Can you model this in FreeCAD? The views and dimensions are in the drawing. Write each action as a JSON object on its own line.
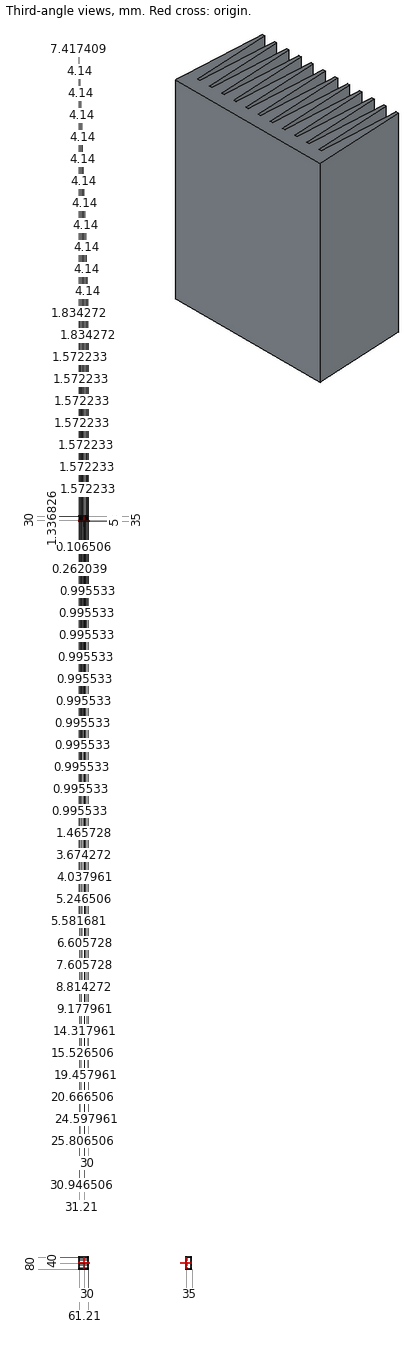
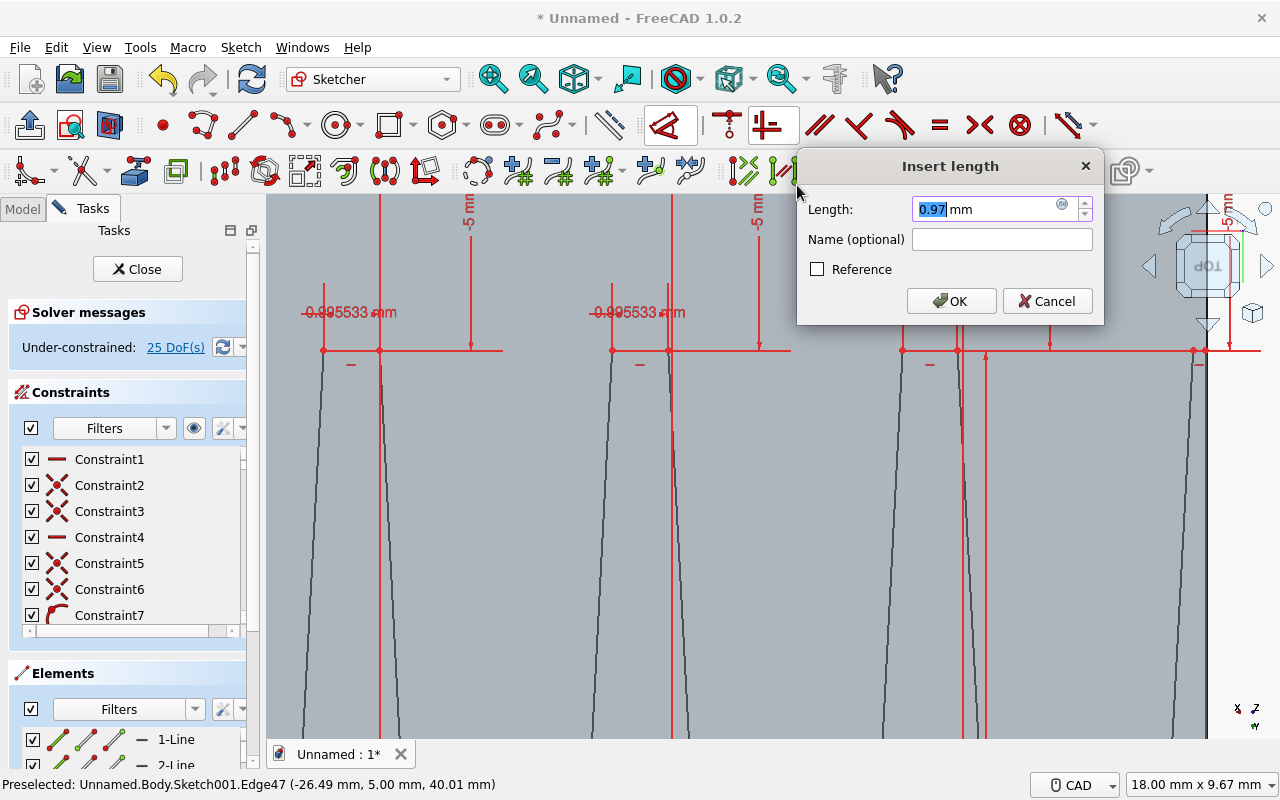
{"action": "type", "text": "0.995533"}
{"action": "key", "text": "Return"}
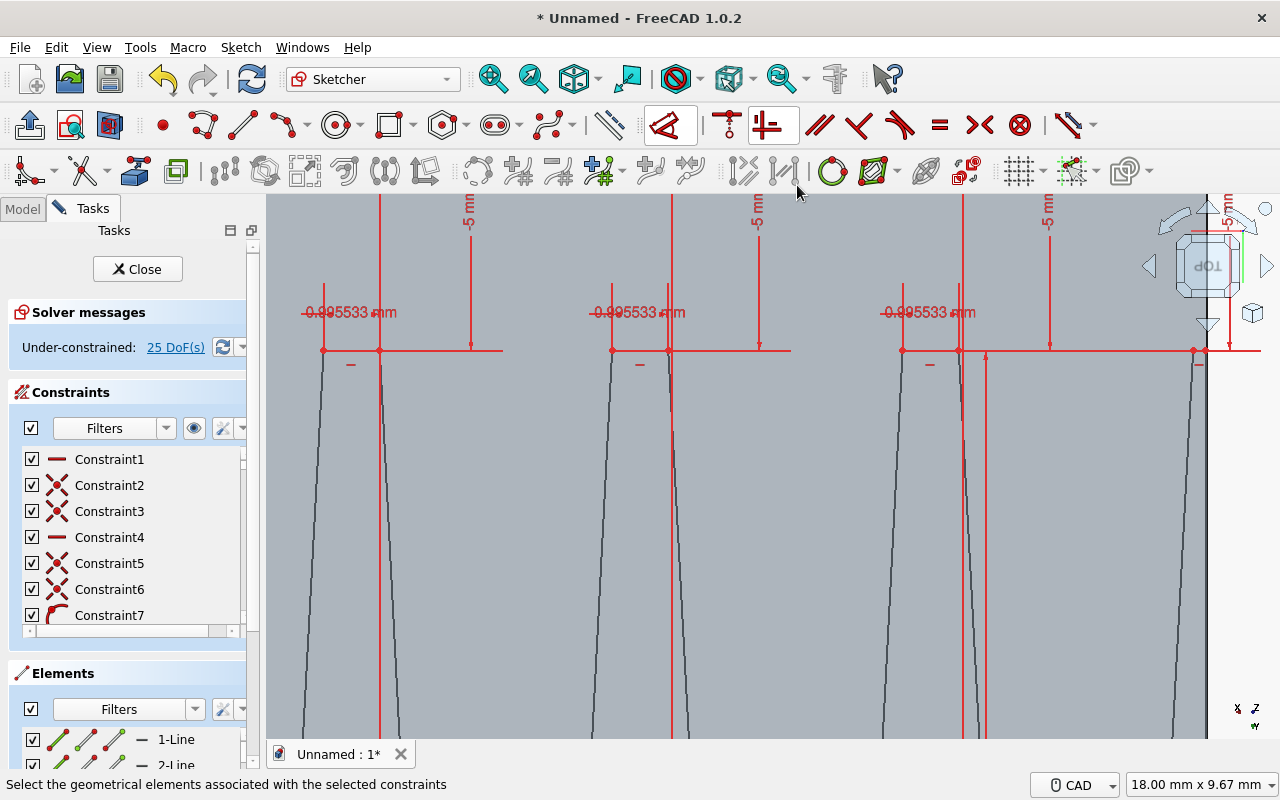
{"action": "scroll", "coordinate": [946, 350], "scroll_direction": "down", "scroll_amount": 9}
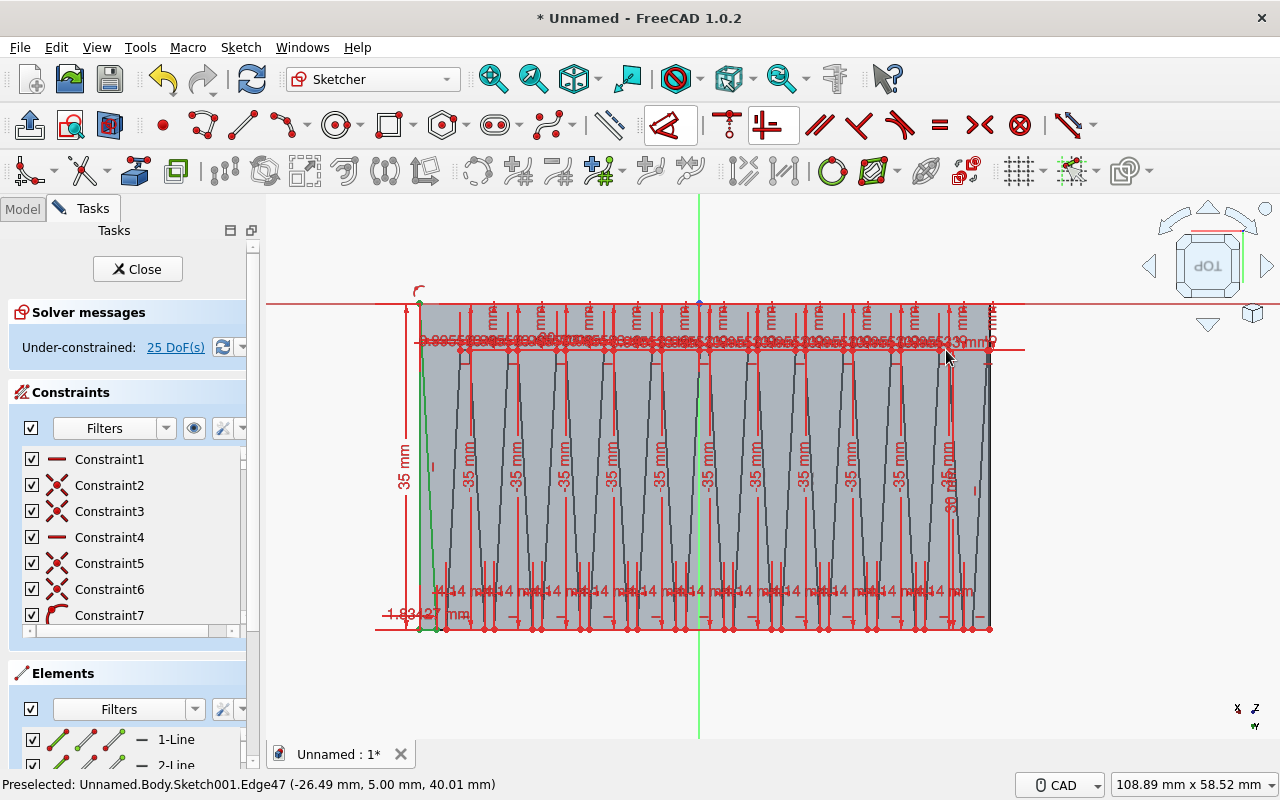
{"action": "scroll", "coordinate": [978, 630], "scroll_direction": "up", "scroll_amount": 5}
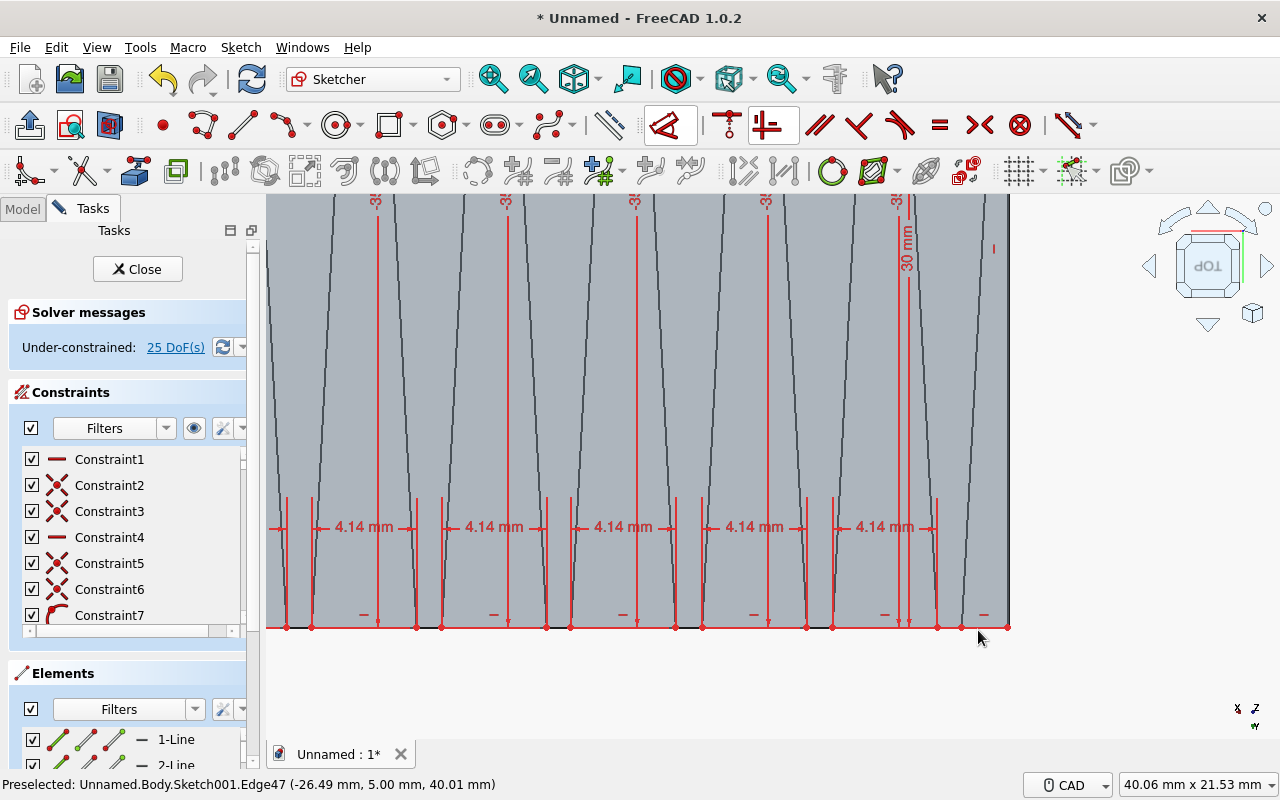
{"action": "left_click", "coordinate": [976, 628]}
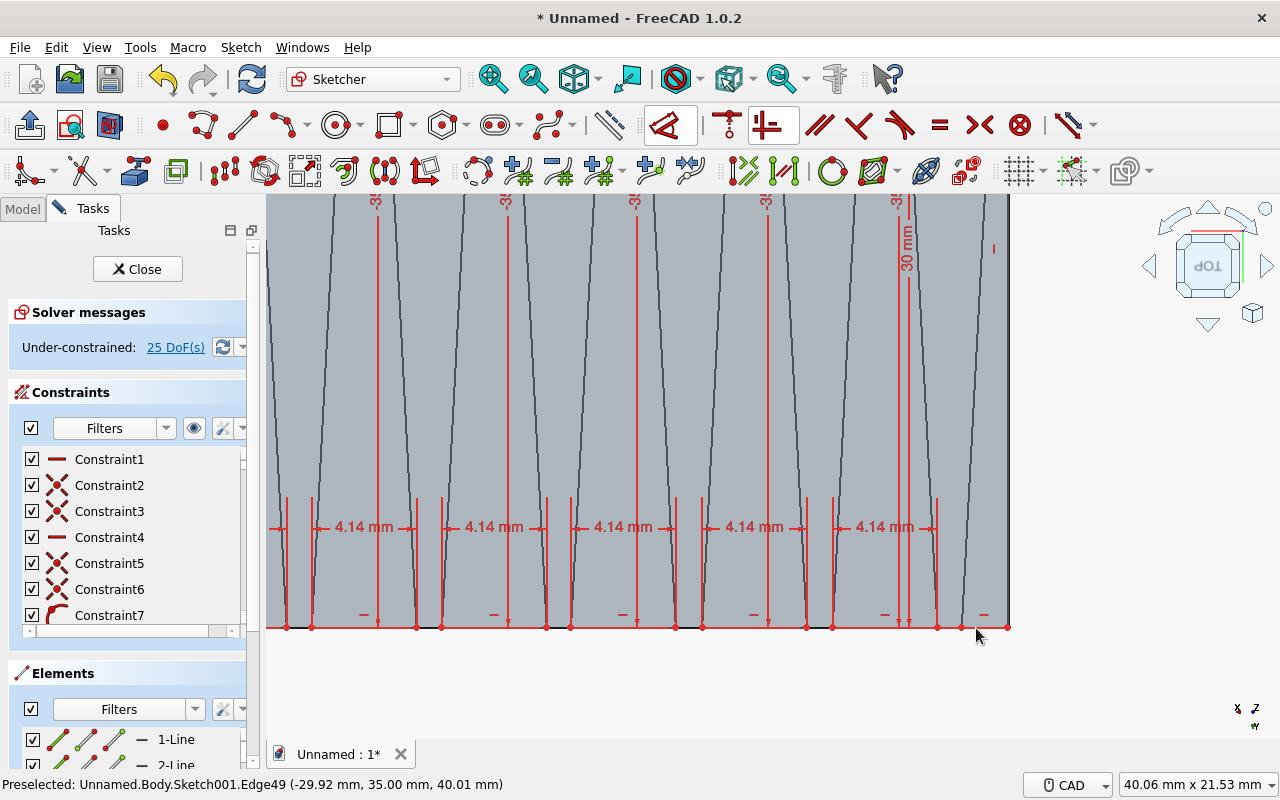
{"action": "left_click", "coordinate": [692, 126]}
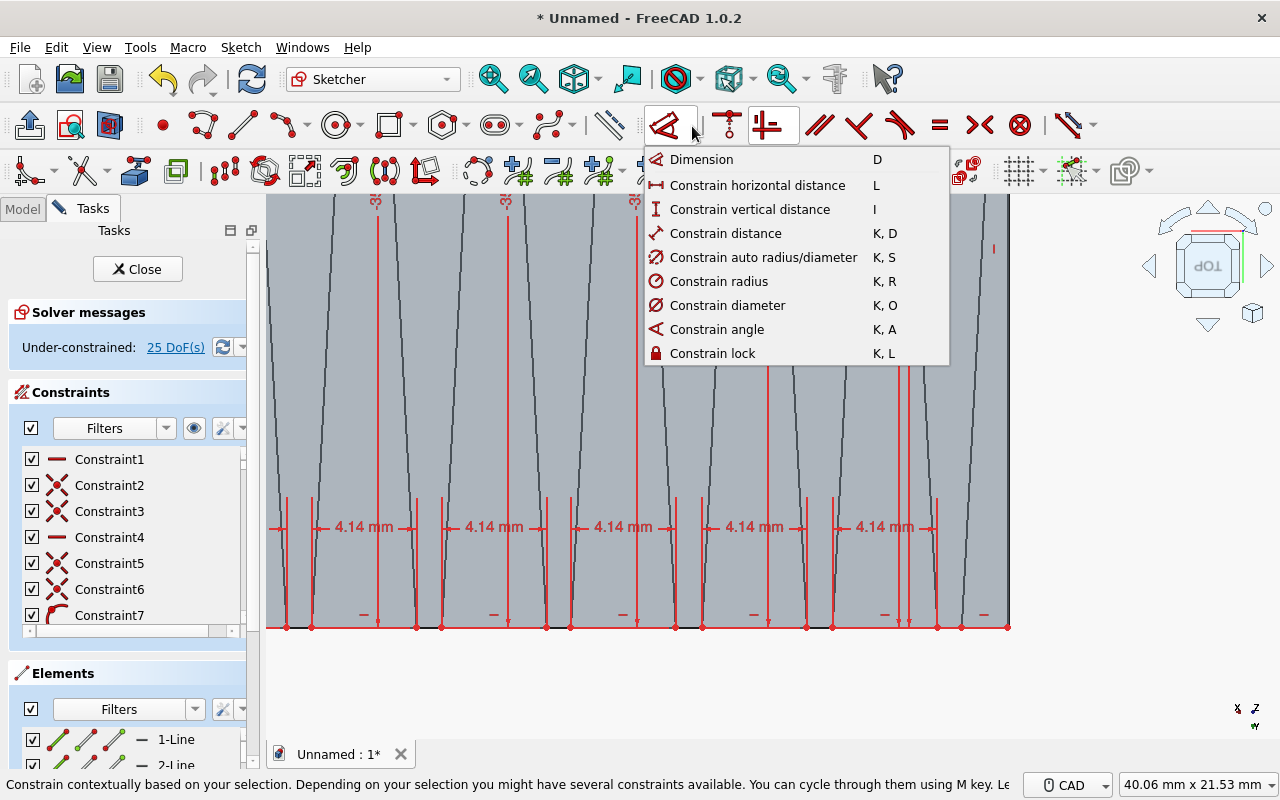
{"action": "left_click", "coordinate": [797, 185]}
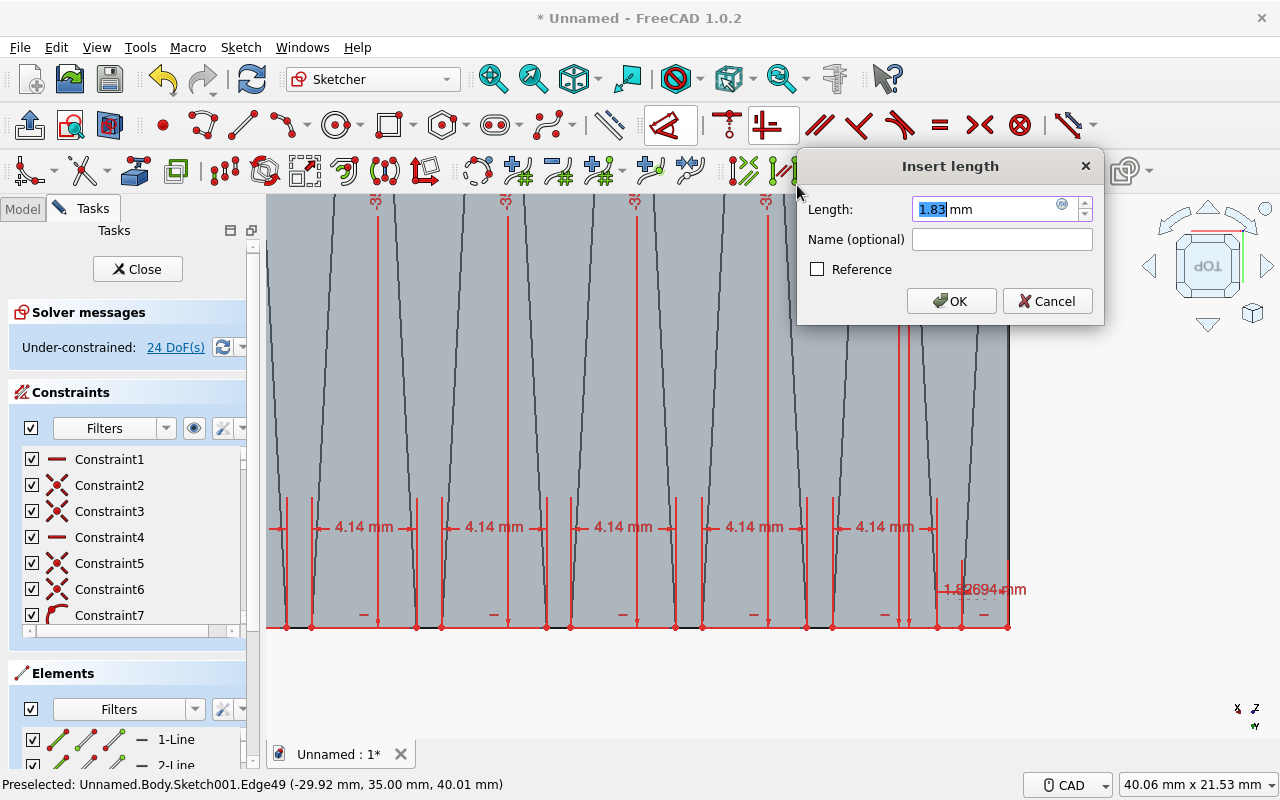
{"action": "type", "text": "1.834272"}
{"action": "key", "text": "Return"}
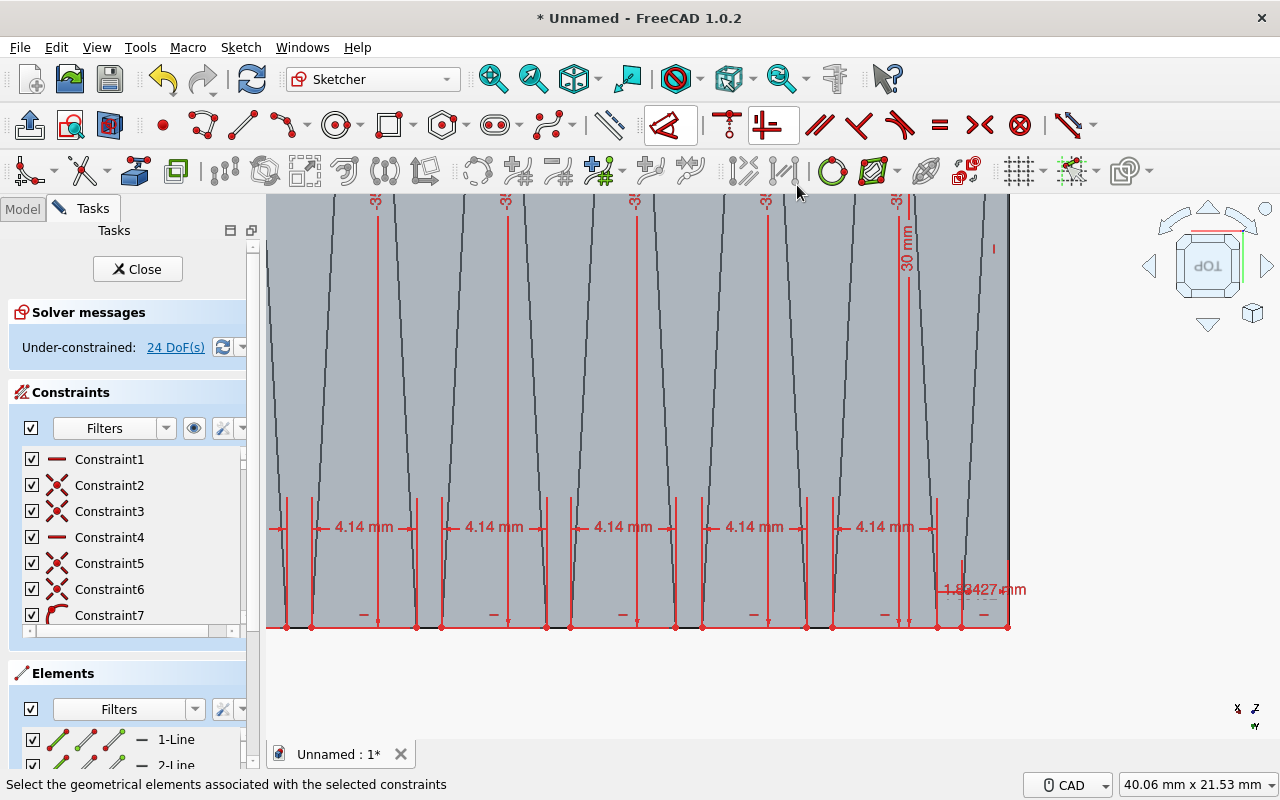
{"action": "scroll", "coordinate": [978, 630], "scroll_direction": "down", "scroll_amount": 5}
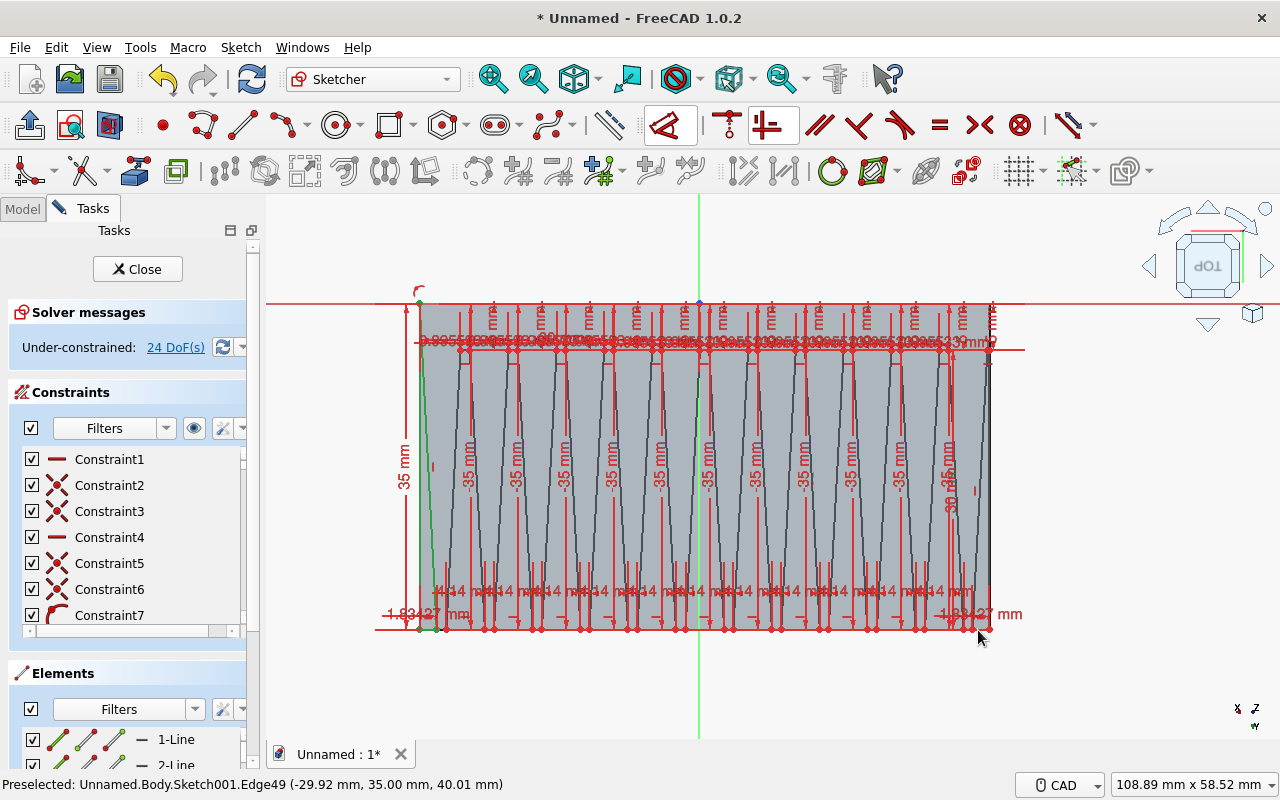
{"action": "scroll", "coordinate": [988, 350], "scroll_direction": "up", "scroll_amount": 14}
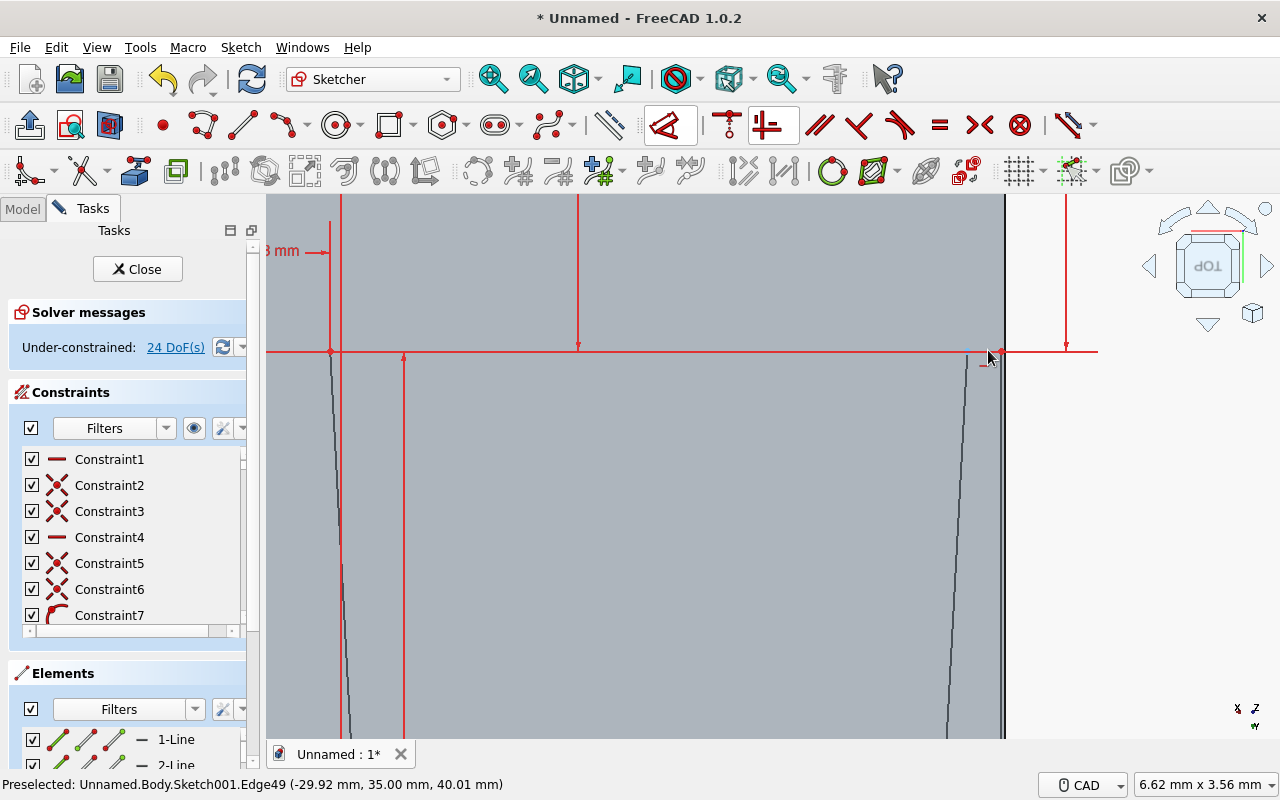
{"action": "left_click", "coordinate": [984, 352]}